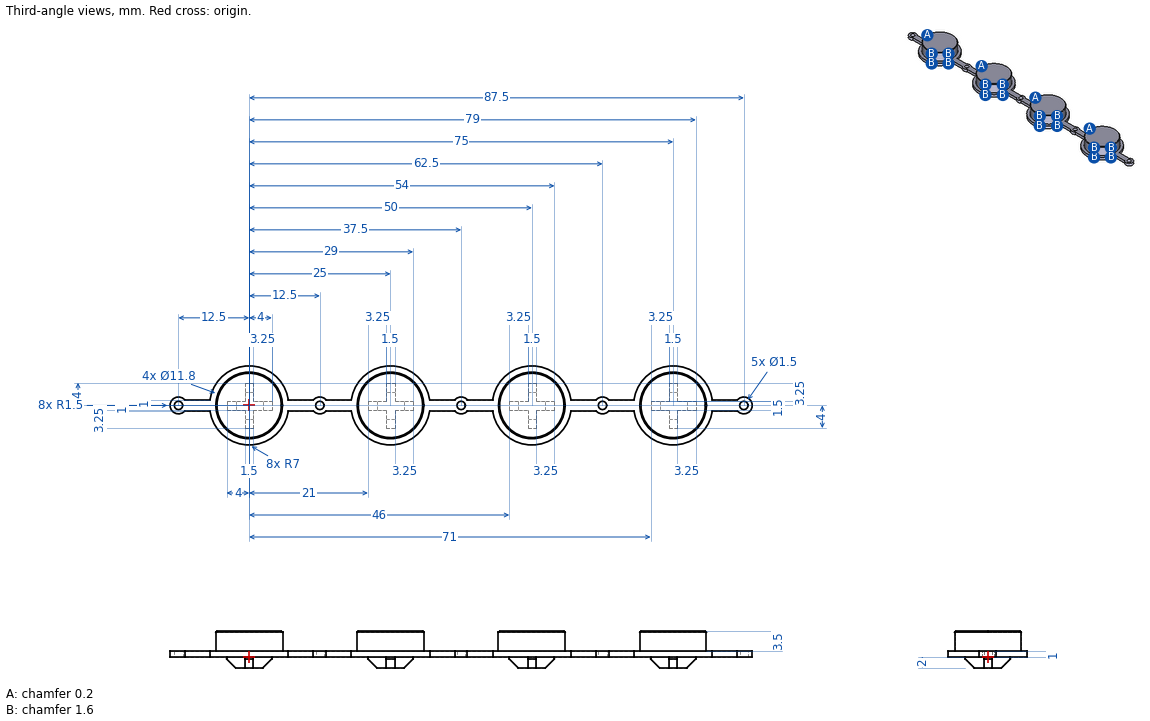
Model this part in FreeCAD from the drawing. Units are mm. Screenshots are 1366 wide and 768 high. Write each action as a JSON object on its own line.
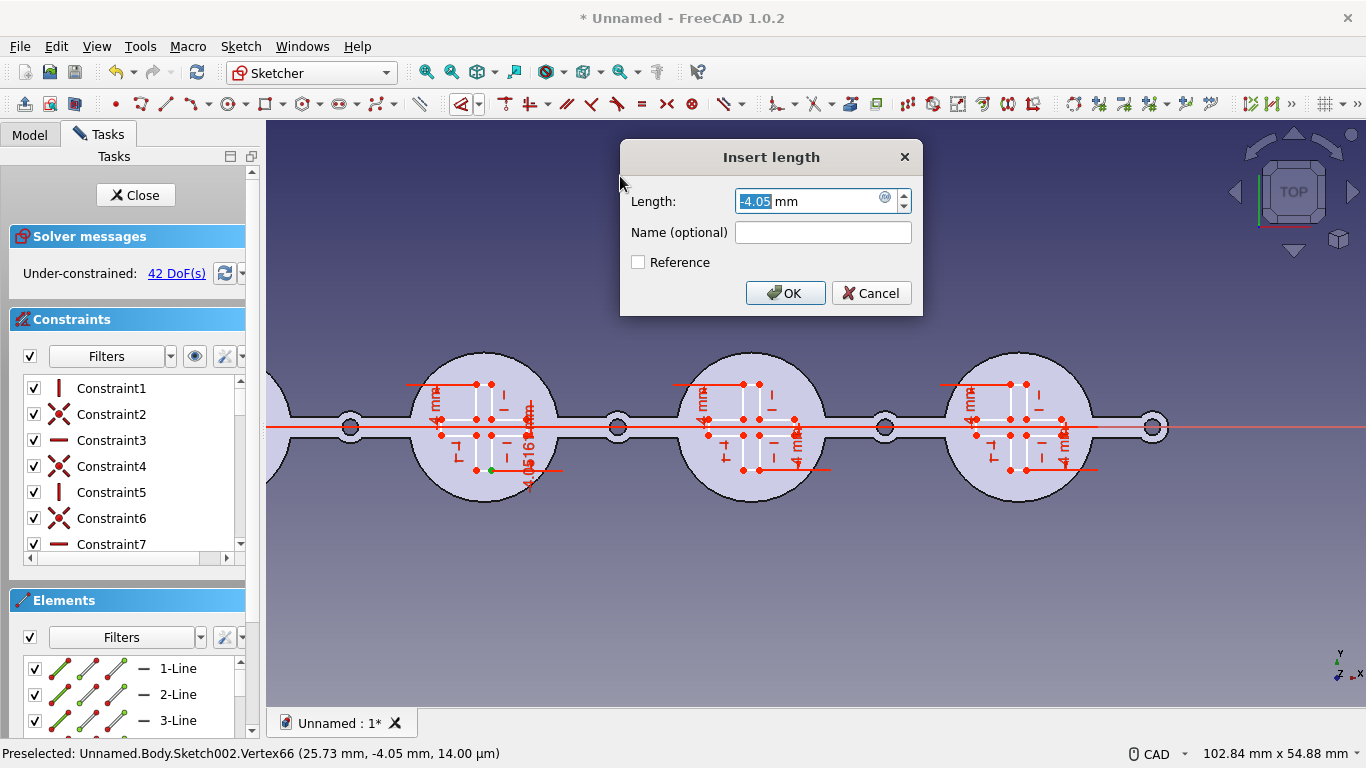
{"action": "type", "text": "-4"}
{"action": "key", "text": "Return"}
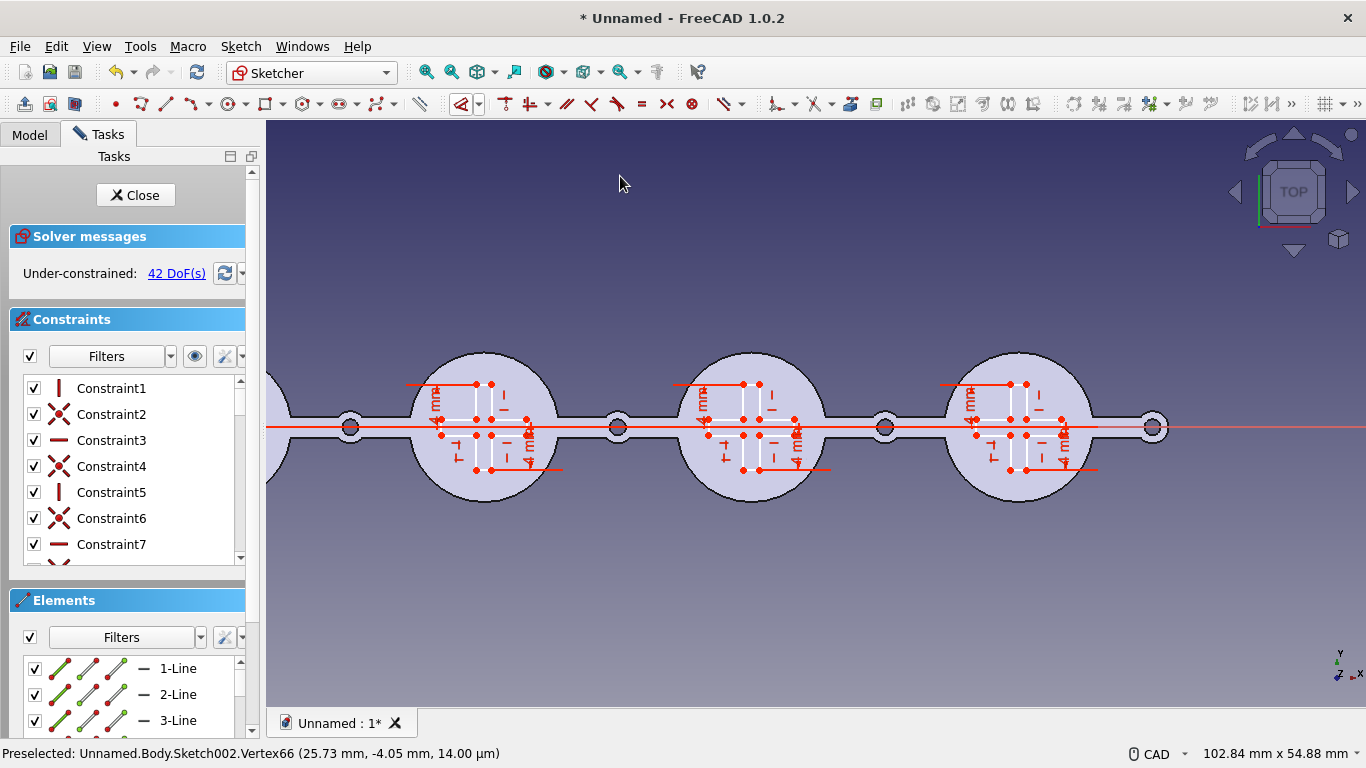
{"action": "scroll", "coordinate": [1011, 385], "scroll_direction": "down", "scroll_amount": 2}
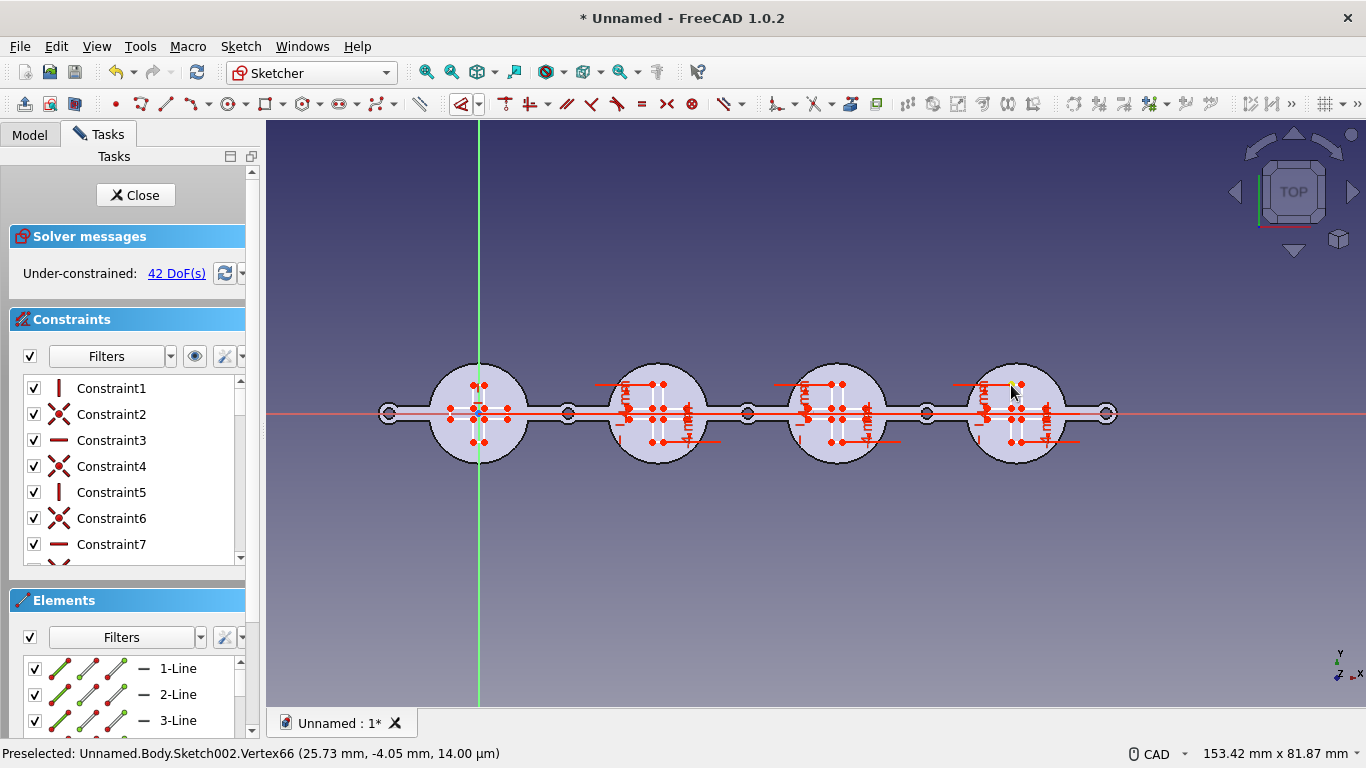
{"action": "scroll", "coordinate": [507, 408], "scroll_direction": "up", "scroll_amount": 2}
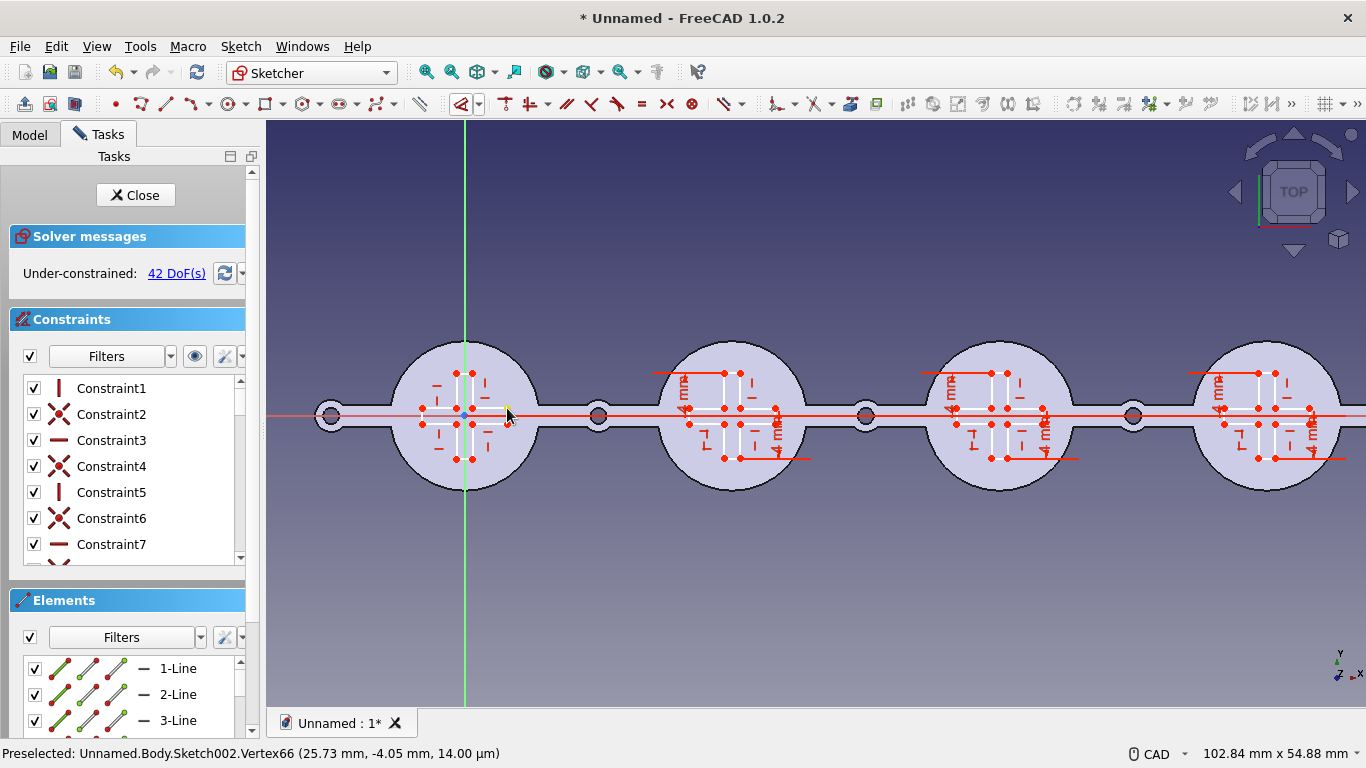
{"action": "left_click", "coordinate": [507, 408]}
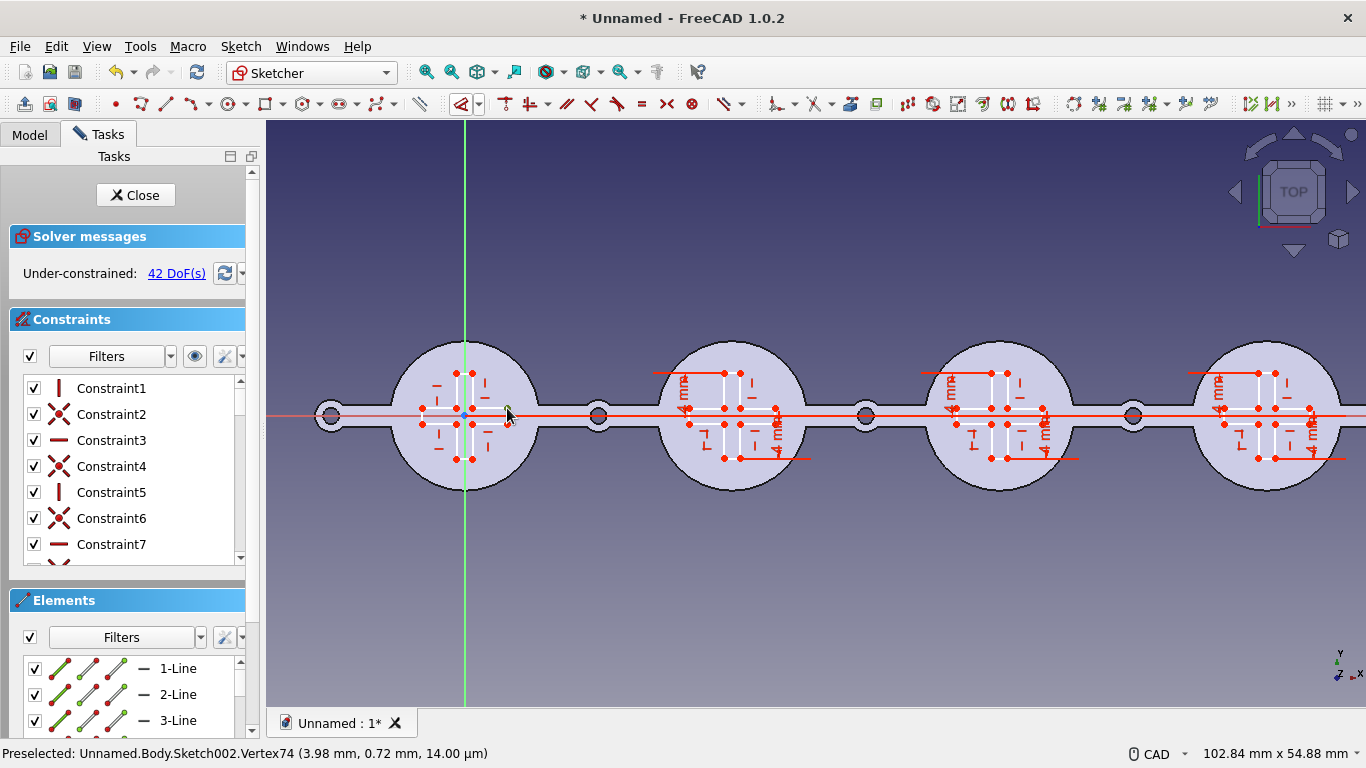
{"action": "left_click", "coordinate": [478, 104]}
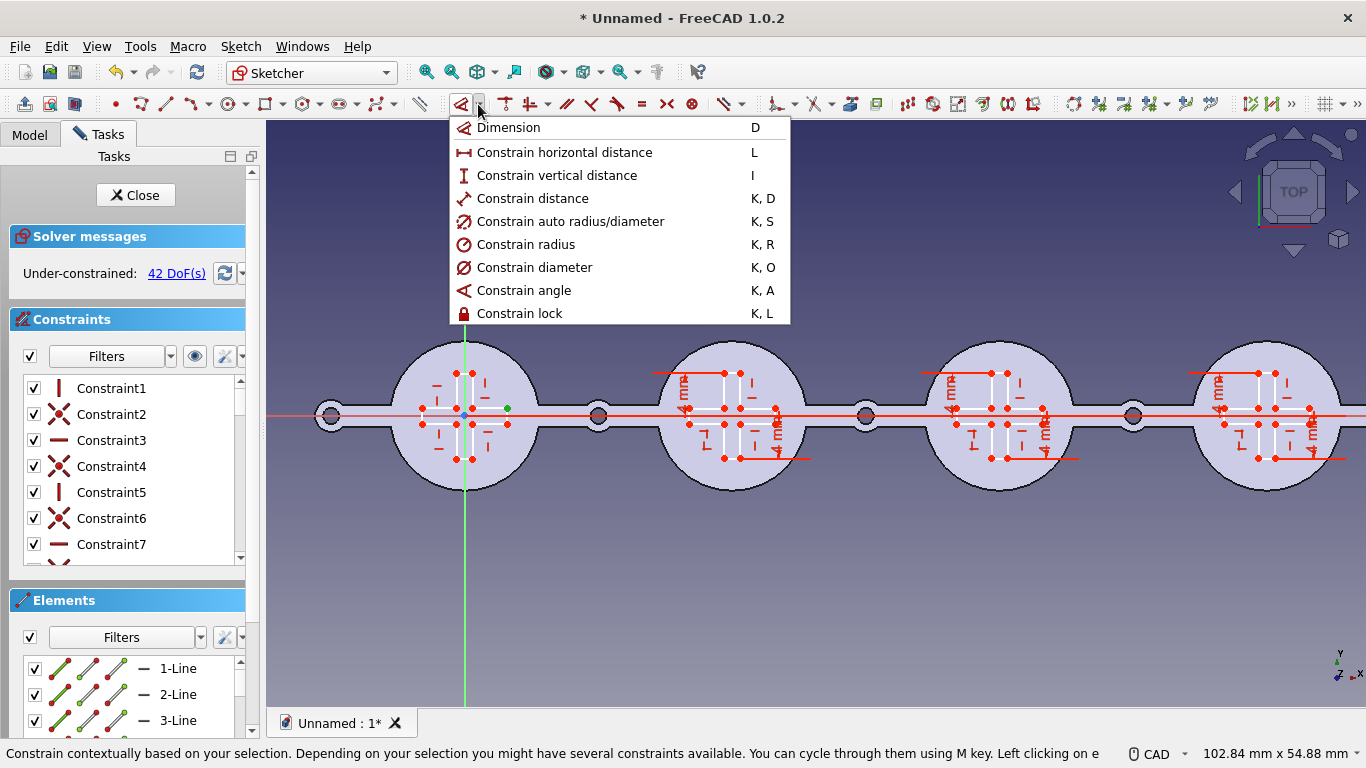
{"action": "left_click", "coordinate": [620, 152]}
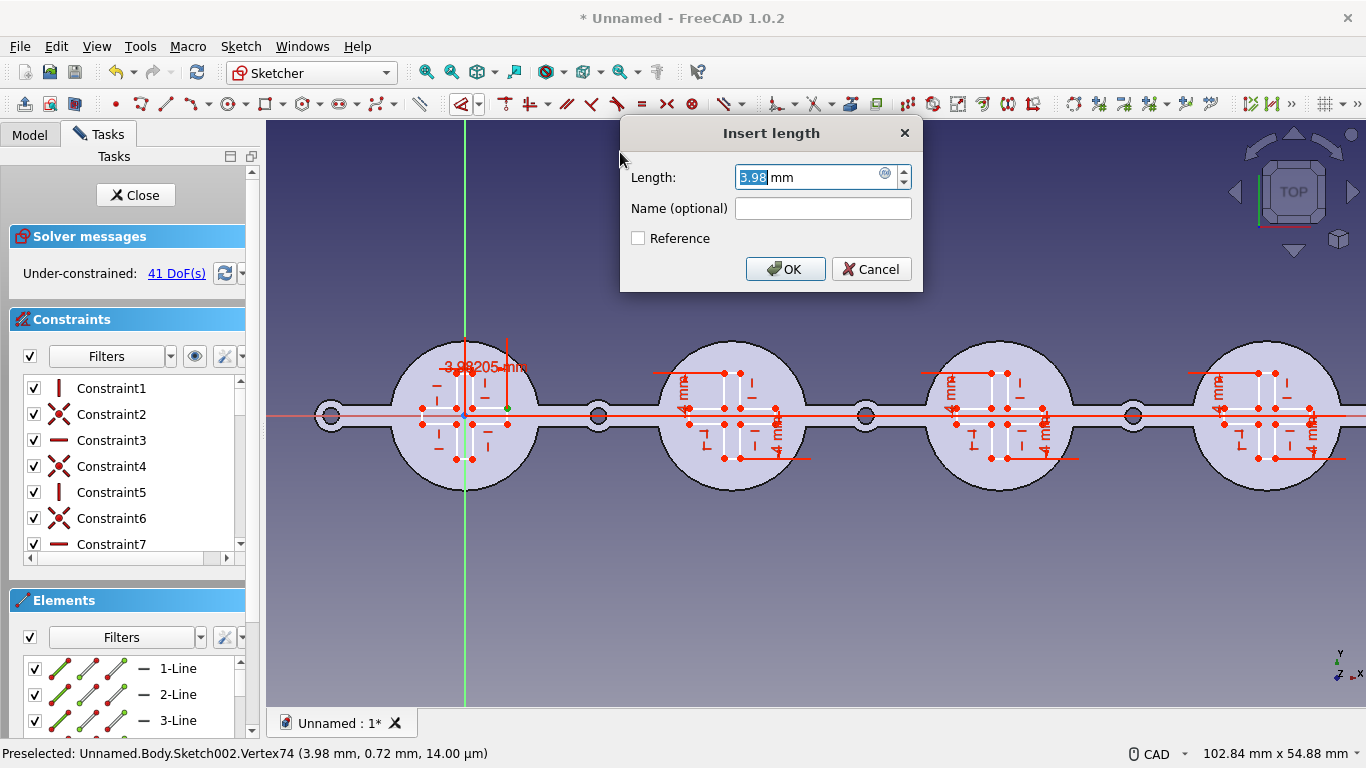
{"action": "type", "text": "4"}
{"action": "key", "text": "Return"}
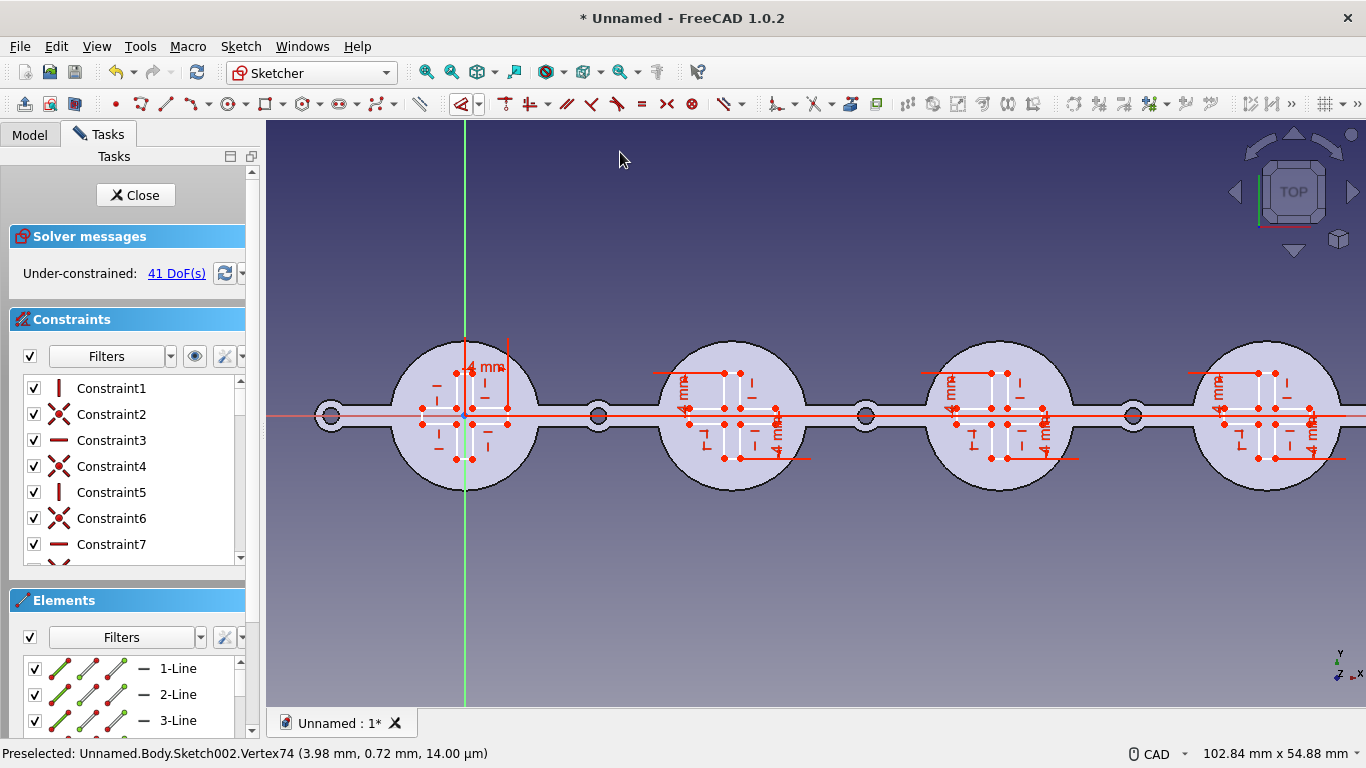
{"action": "left_click", "coordinate": [473, 459]}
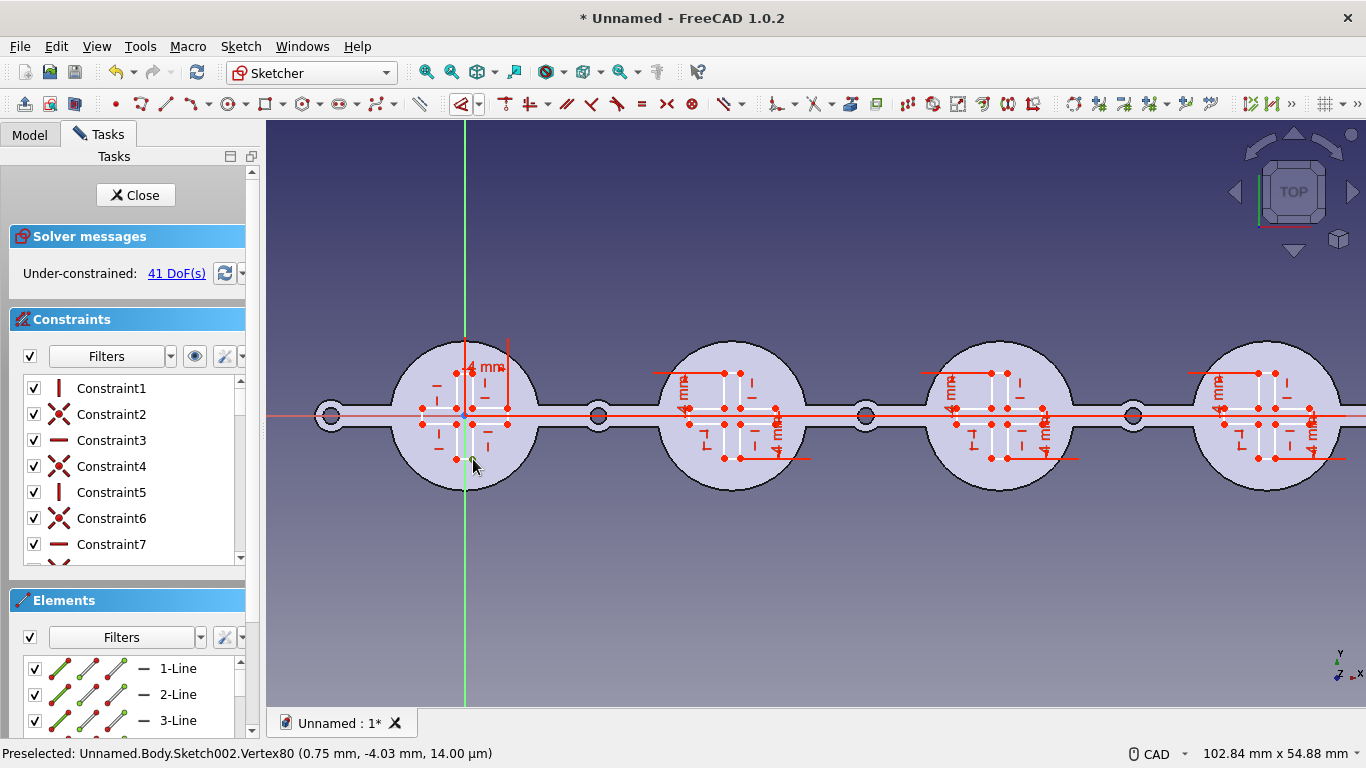
{"action": "key", "text": "i"}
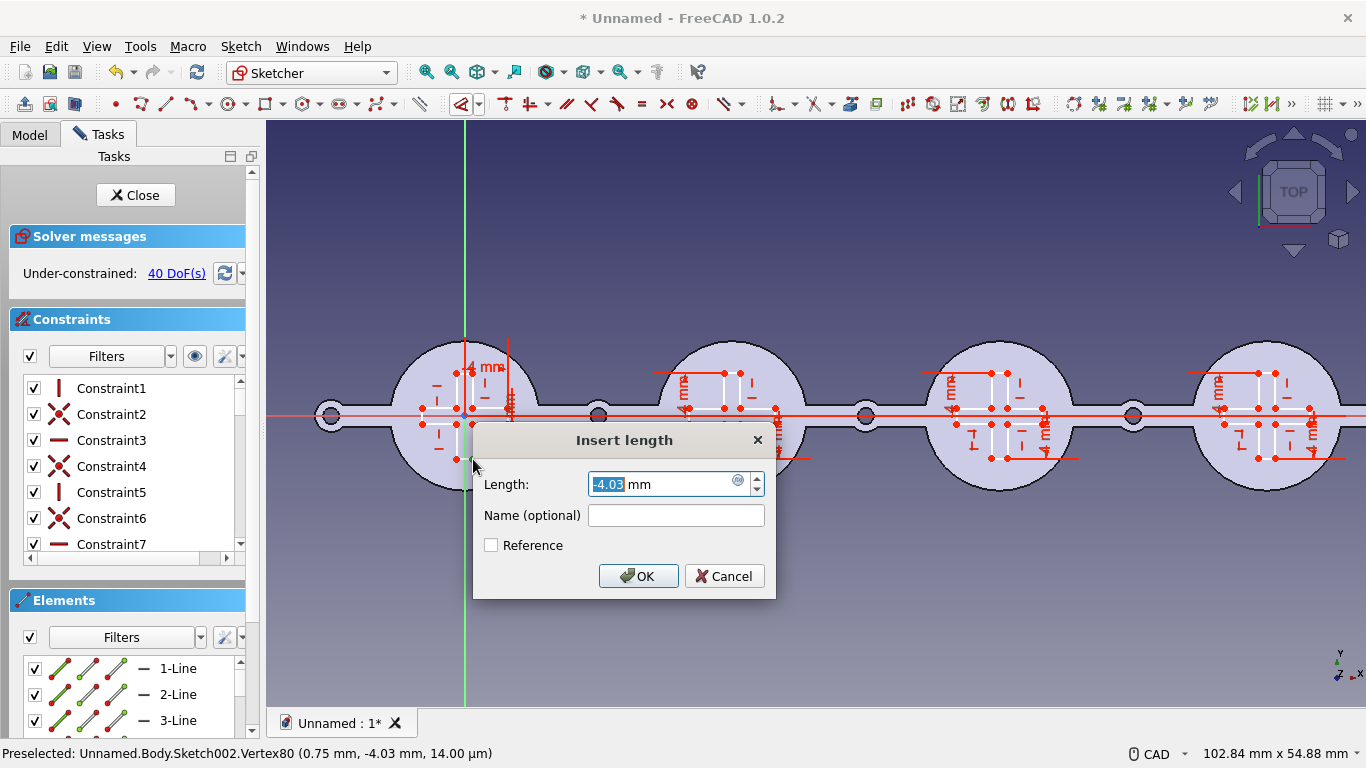
{"action": "type", "text": "-4"}
{"action": "key", "text": "Return"}